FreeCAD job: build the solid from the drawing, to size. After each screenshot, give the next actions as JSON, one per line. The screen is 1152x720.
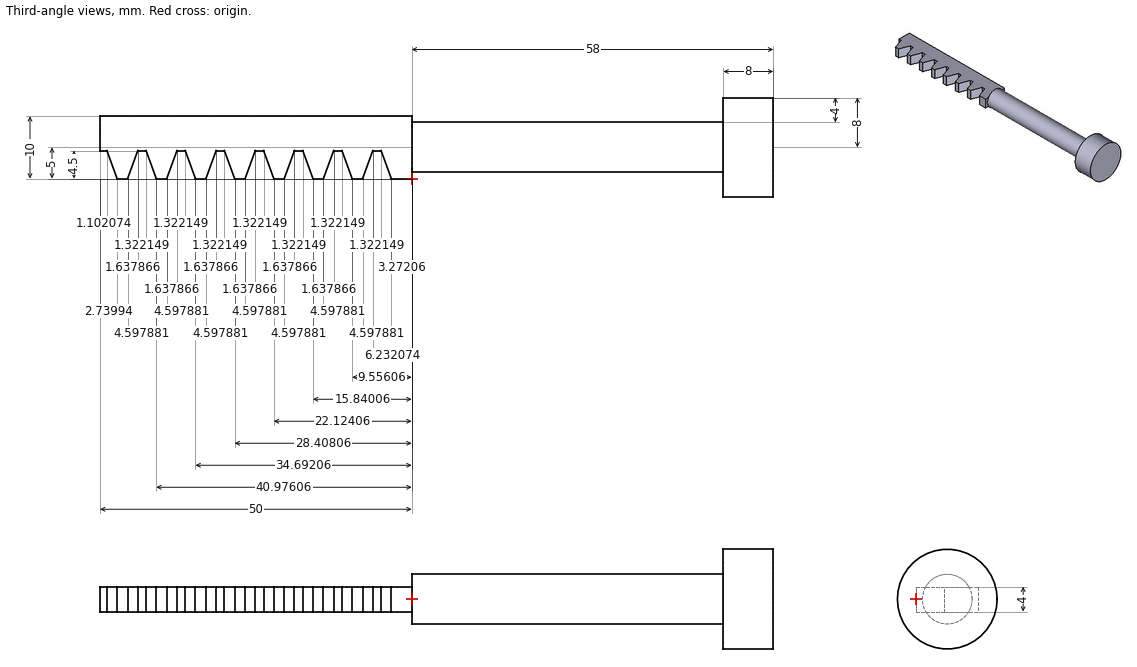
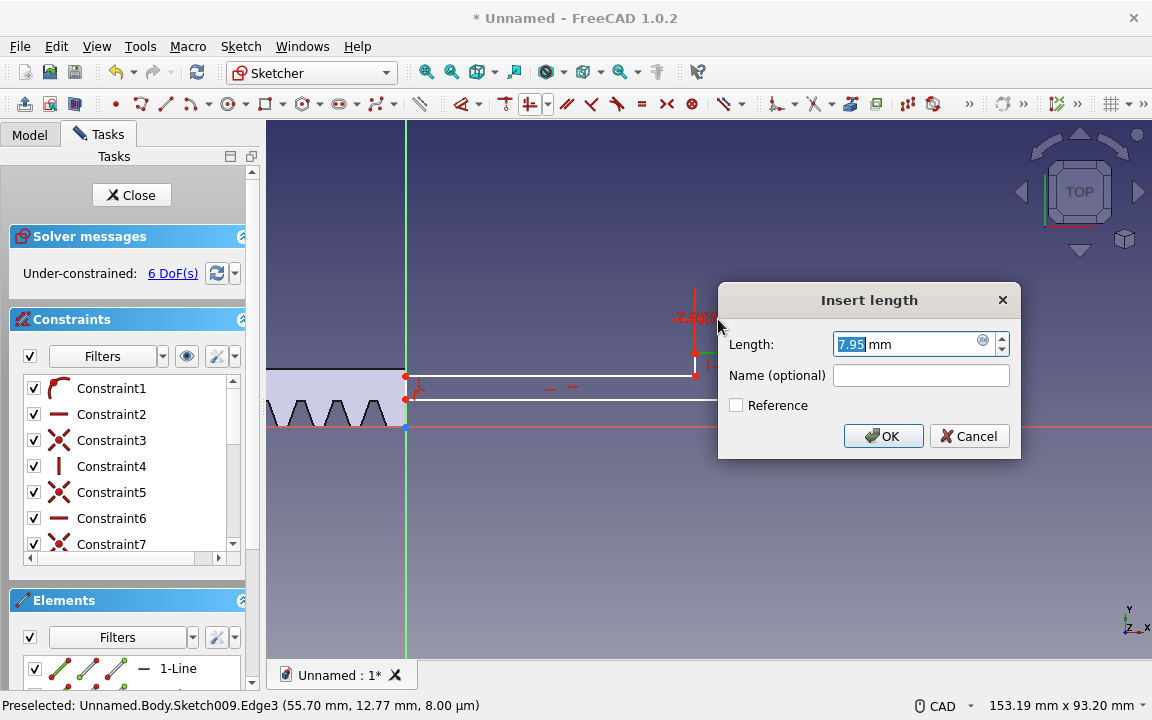
{"action": "type", "text": "8"}
{"action": "key", "text": "Return"}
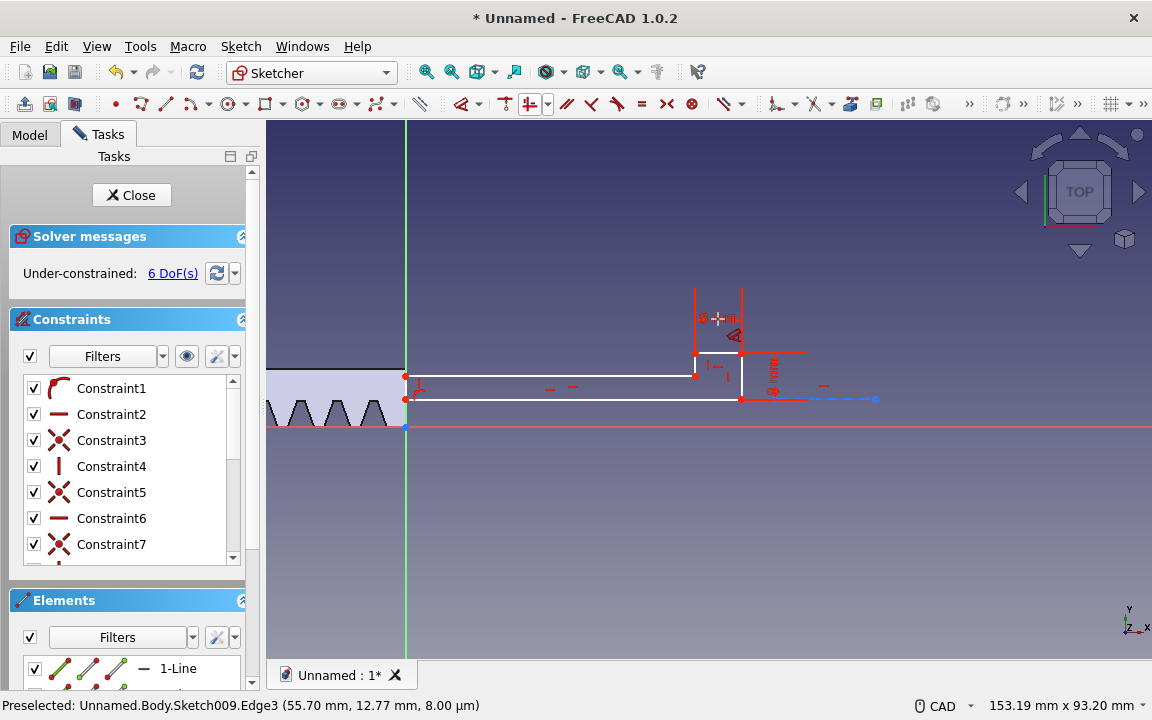
{"action": "scroll", "coordinate": [695, 363], "scroll_direction": "up", "scroll_amount": 3}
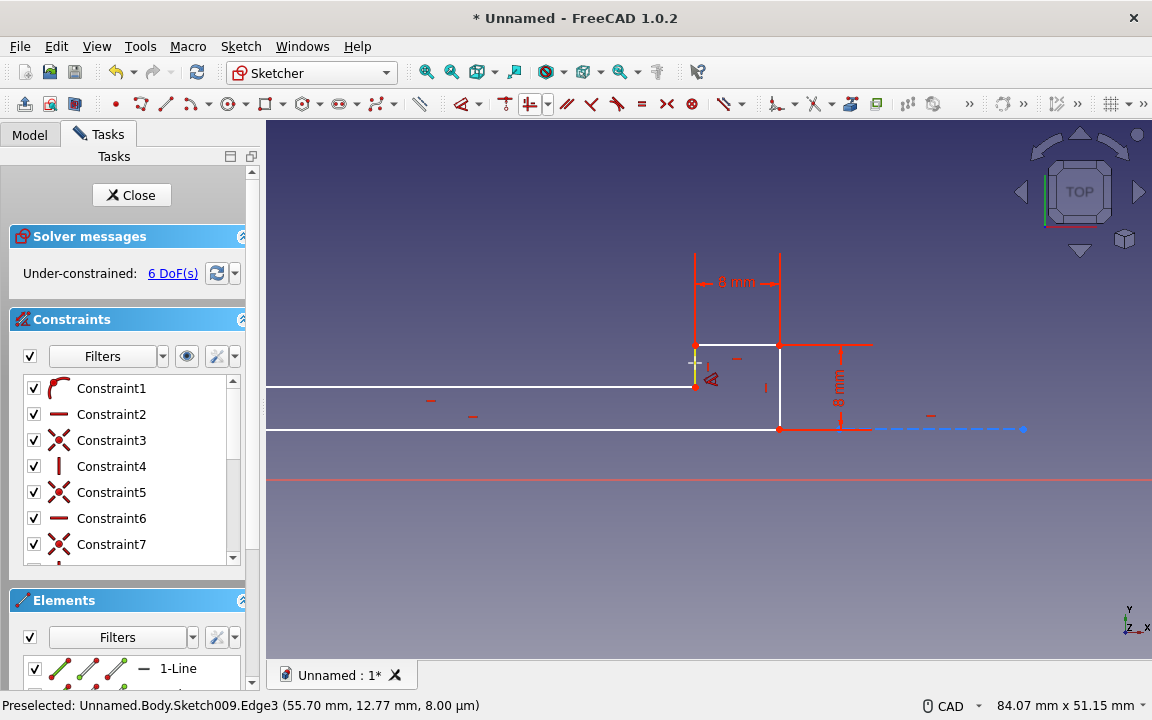
{"action": "left_click", "coordinate": [695, 362]}
{"action": "left_click", "coordinate": [729, 366]}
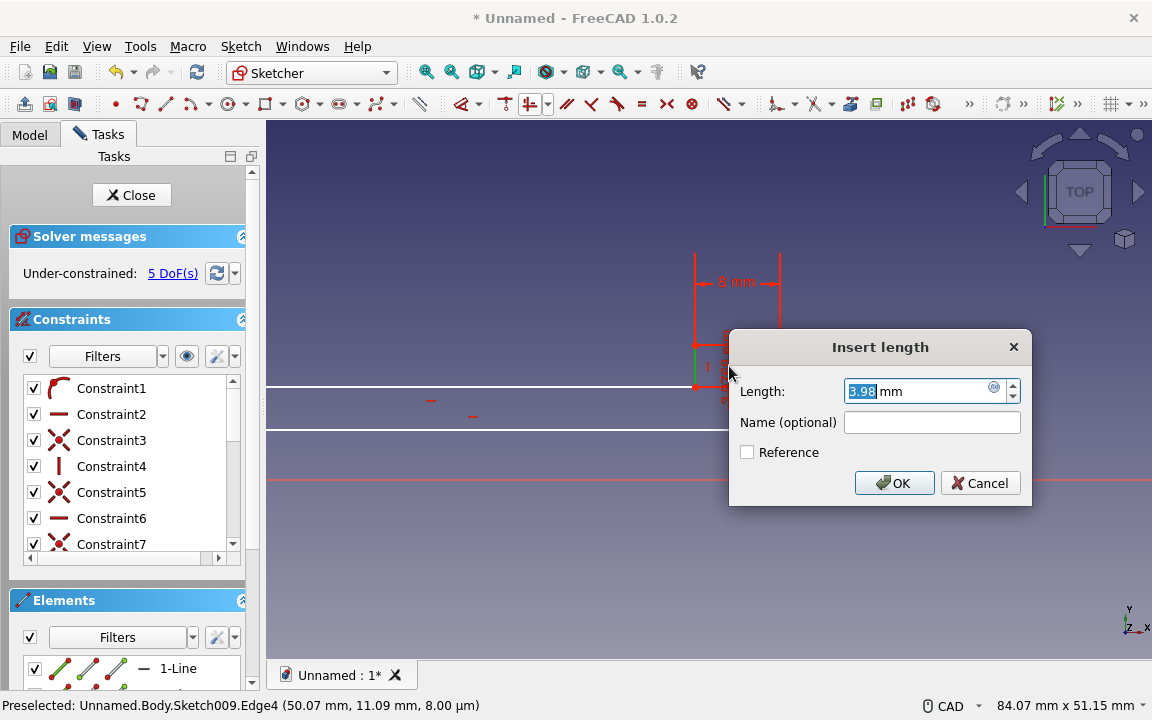
{"action": "type", "text": "4"}
{"action": "key", "text": "Return"}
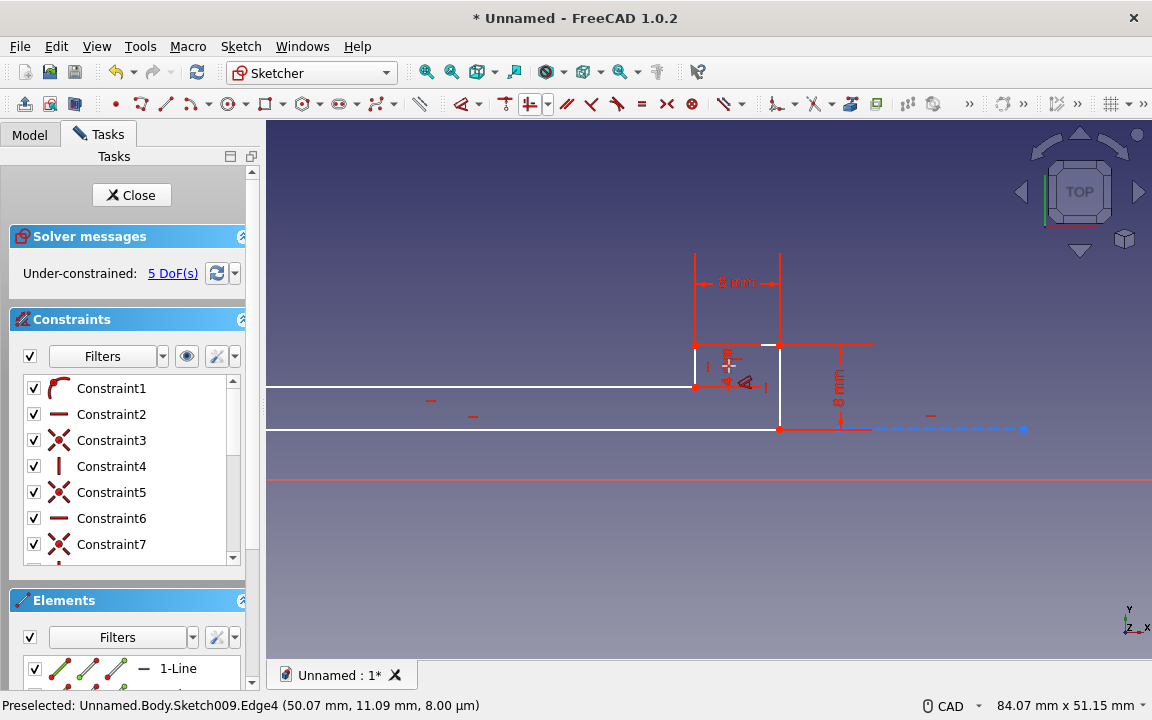
{"action": "left_click", "coordinate": [351, 430]}
{"action": "left_click", "coordinate": [537, 464]}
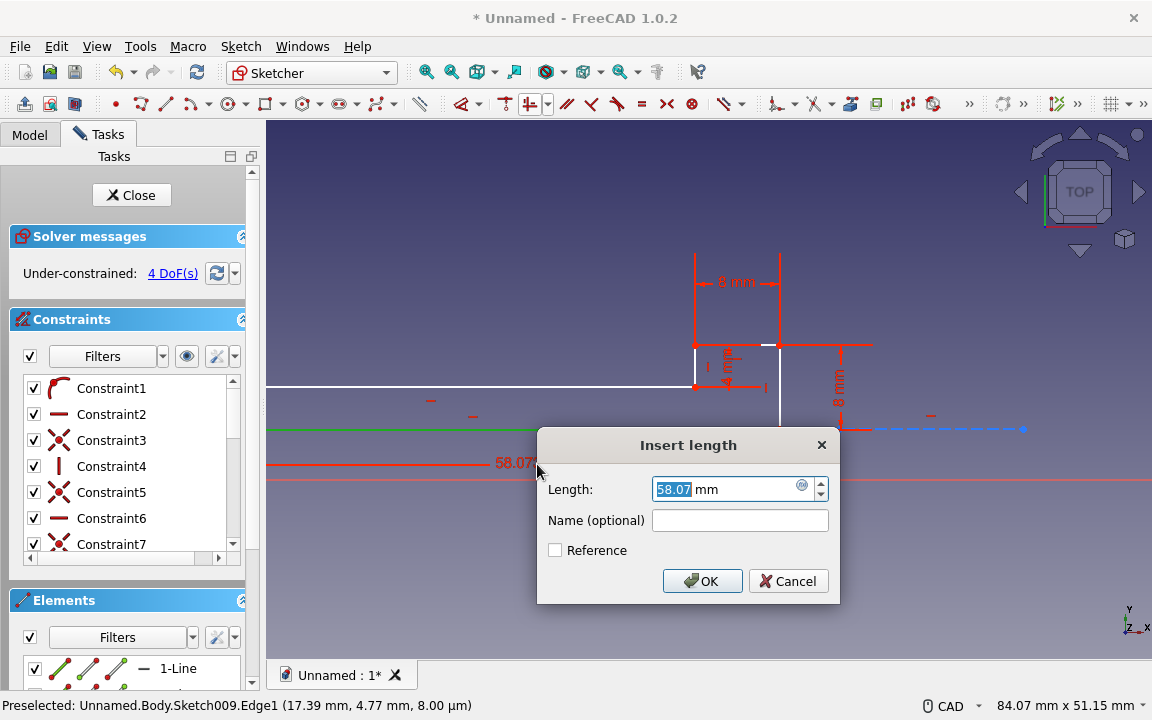
{"action": "type", "text": "58"}
{"action": "key", "text": "Return"}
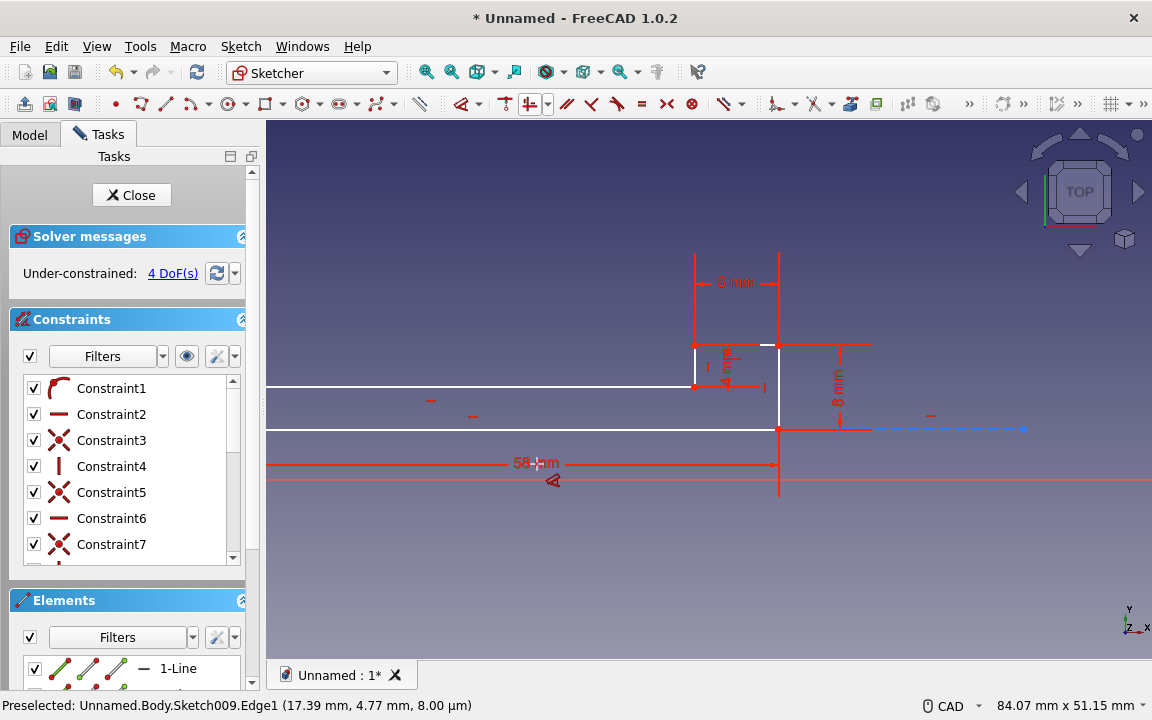
{"action": "scroll", "coordinate": [695, 363], "scroll_direction": "down", "scroll_amount": 3}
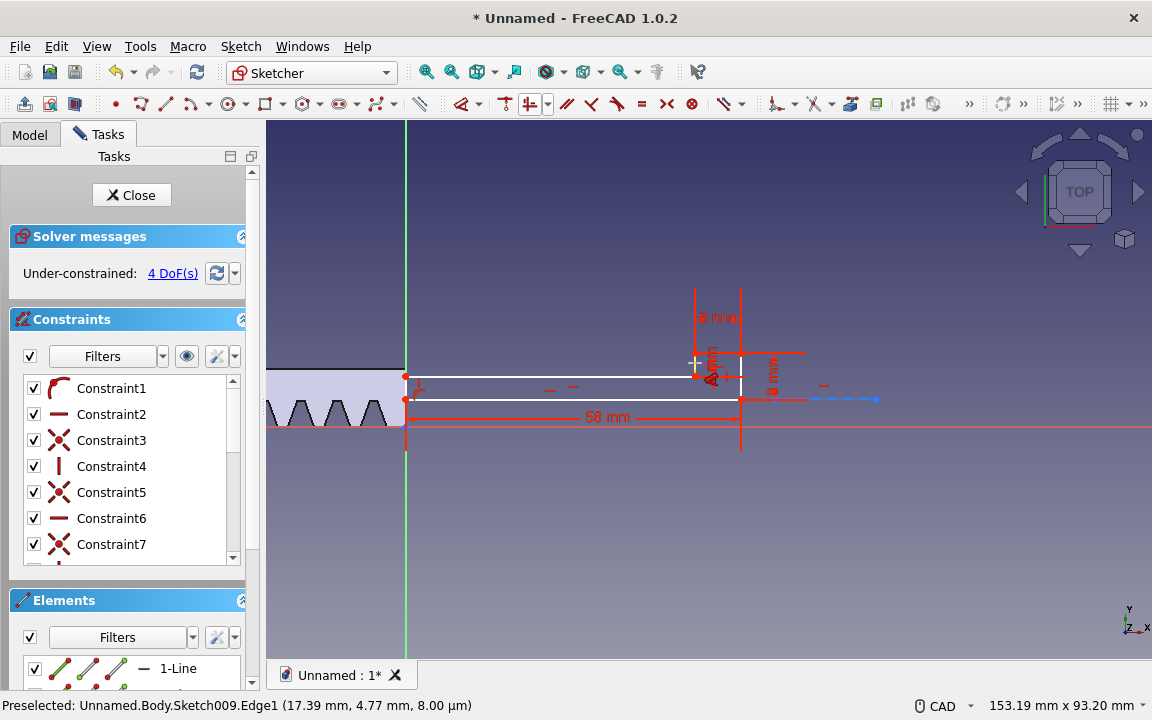
{"action": "scroll", "coordinate": [406, 400], "scroll_direction": "up", "scroll_amount": 2}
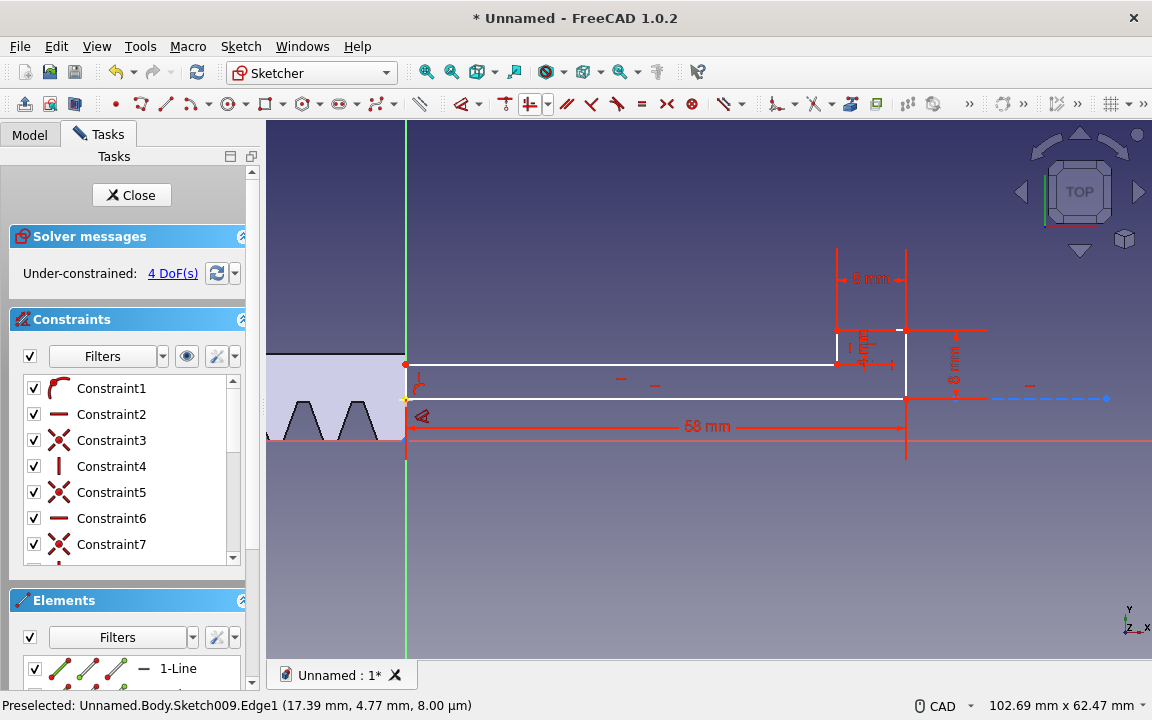
{"action": "left_click", "coordinate": [406, 399]}
{"action": "left_click", "coordinate": [372, 420]}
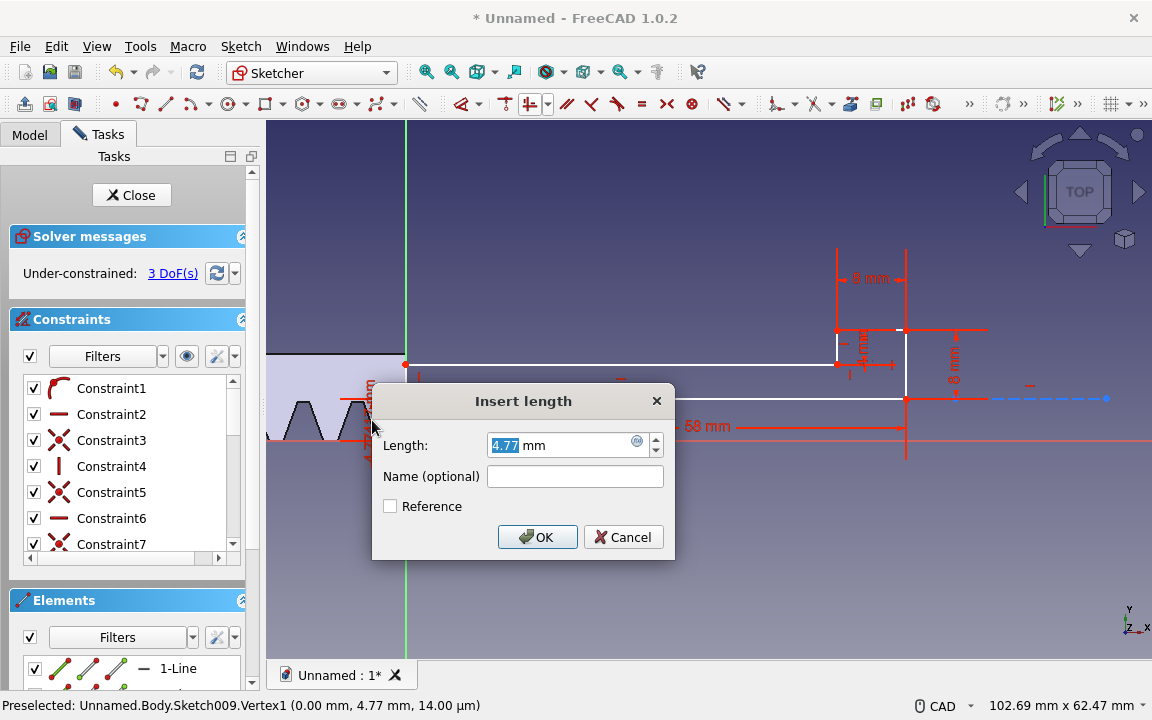
{"action": "type", "text": "5"}
{"action": "key", "text": "Return"}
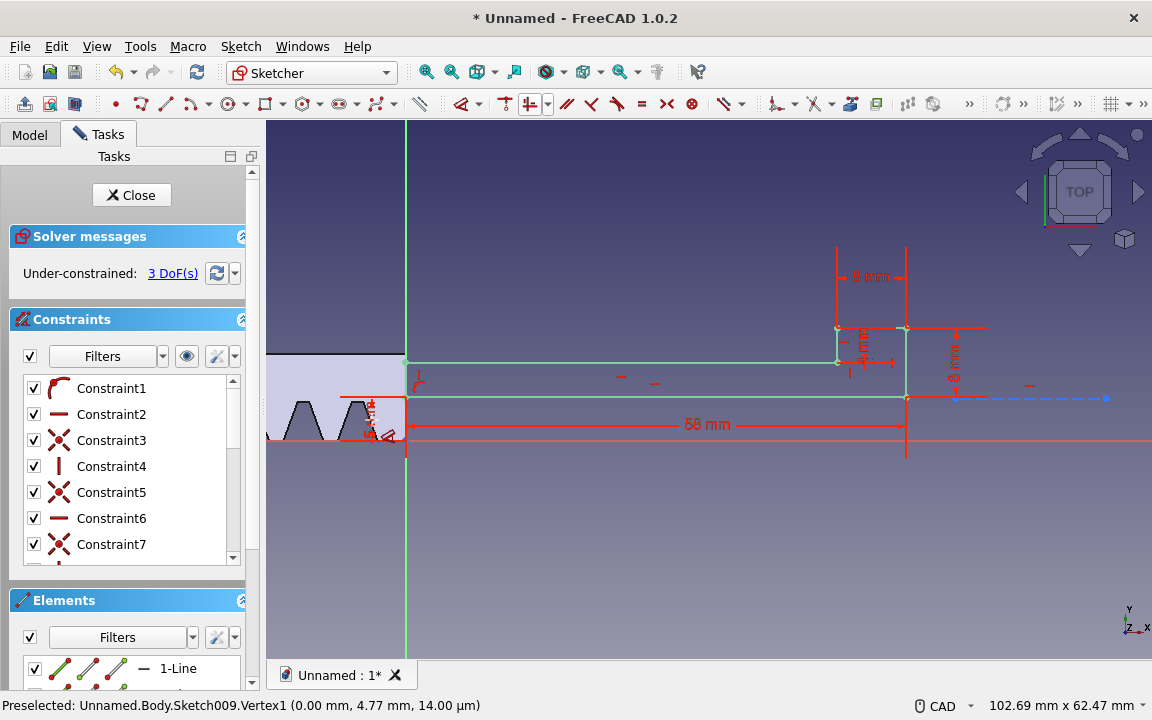
{"action": "left_click", "coordinate": [956, 399]}
{"action": "left_click", "coordinate": [300, 420]}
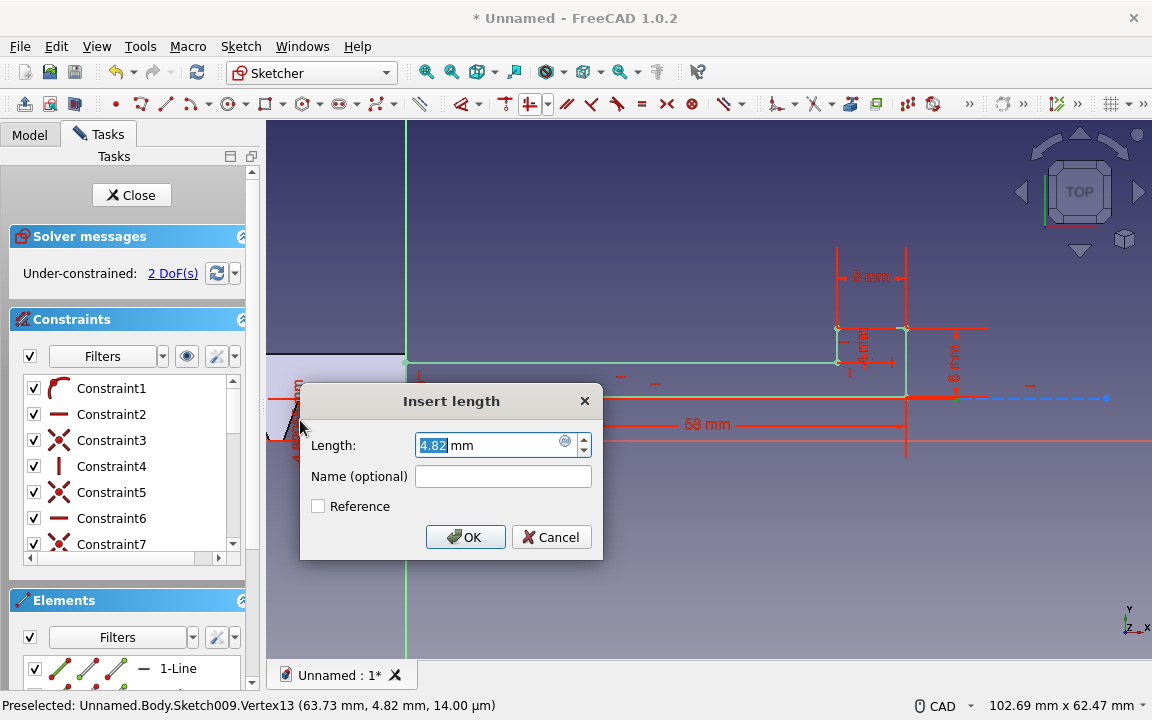
{"action": "type", "text": "5"}
{"action": "key", "text": "Return"}
{"action": "key", "text": "Escape"}